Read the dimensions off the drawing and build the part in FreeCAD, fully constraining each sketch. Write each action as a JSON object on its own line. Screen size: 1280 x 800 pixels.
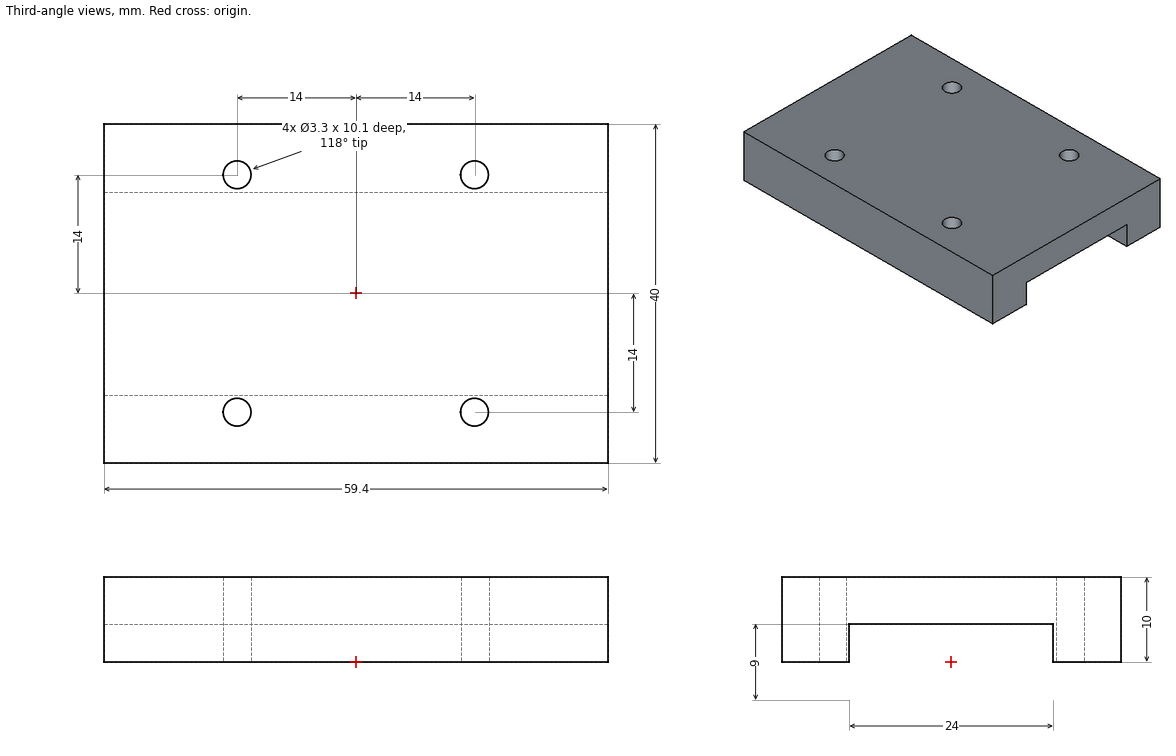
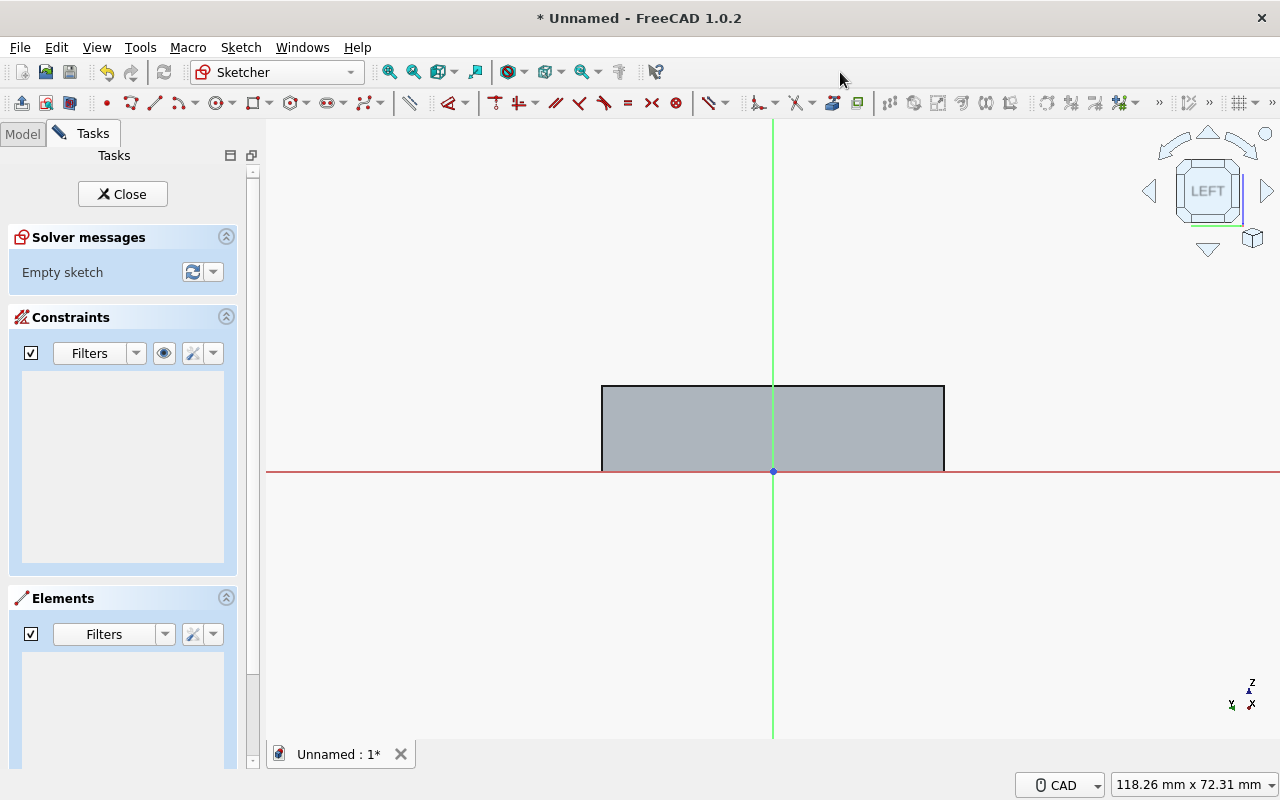
{"action": "scroll", "coordinate": [813, 497], "scroll_direction": "up", "scroll_amount": 5}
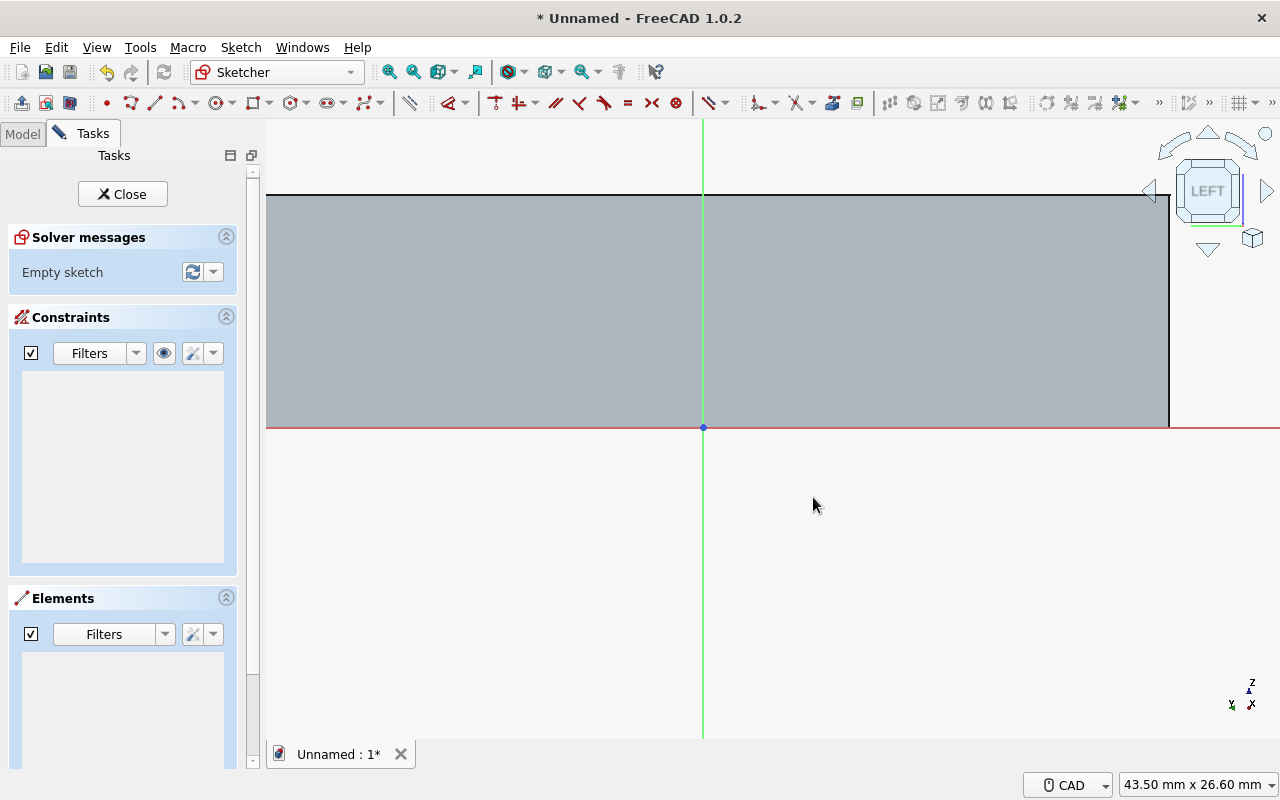
{"action": "key", "text": "g v"}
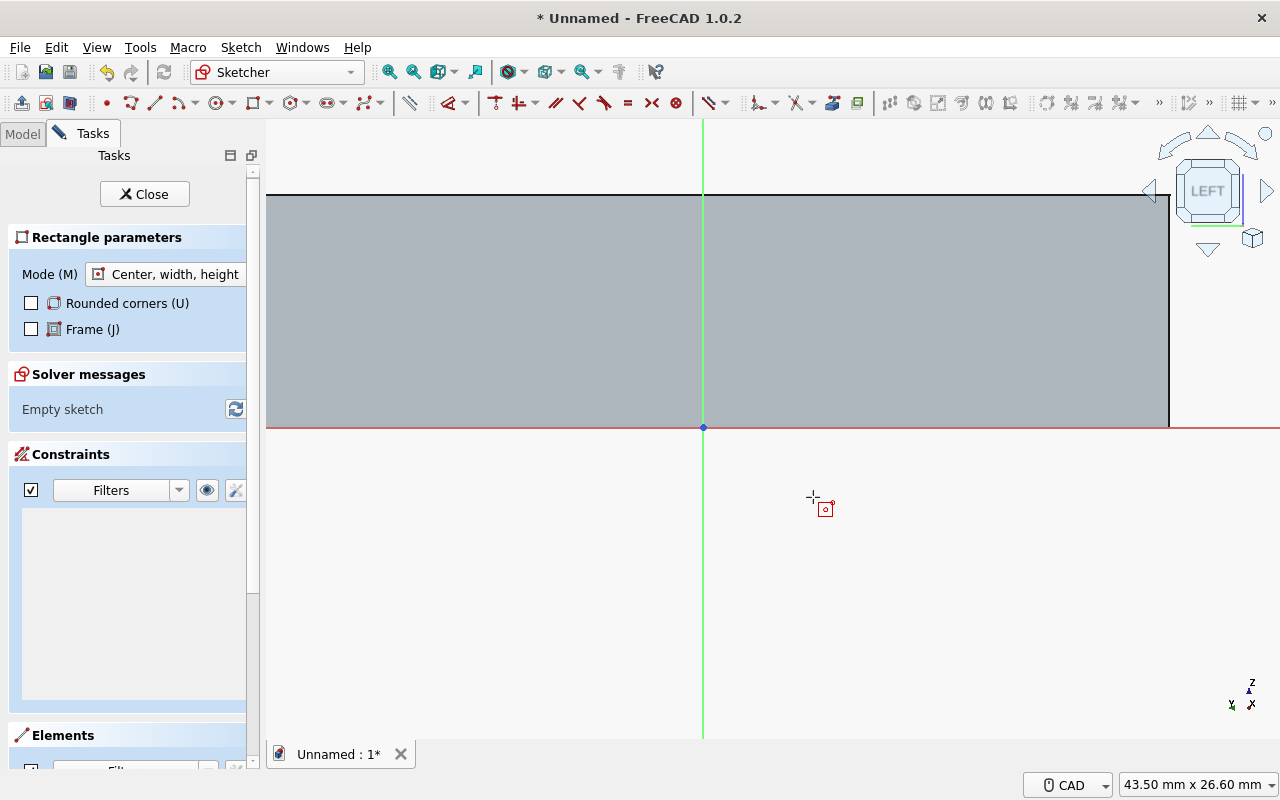
{"action": "left_click", "coordinate": [703, 428]}
{"action": "left_click", "coordinate": [983, 323]}
{"action": "key", "text": "Escape"}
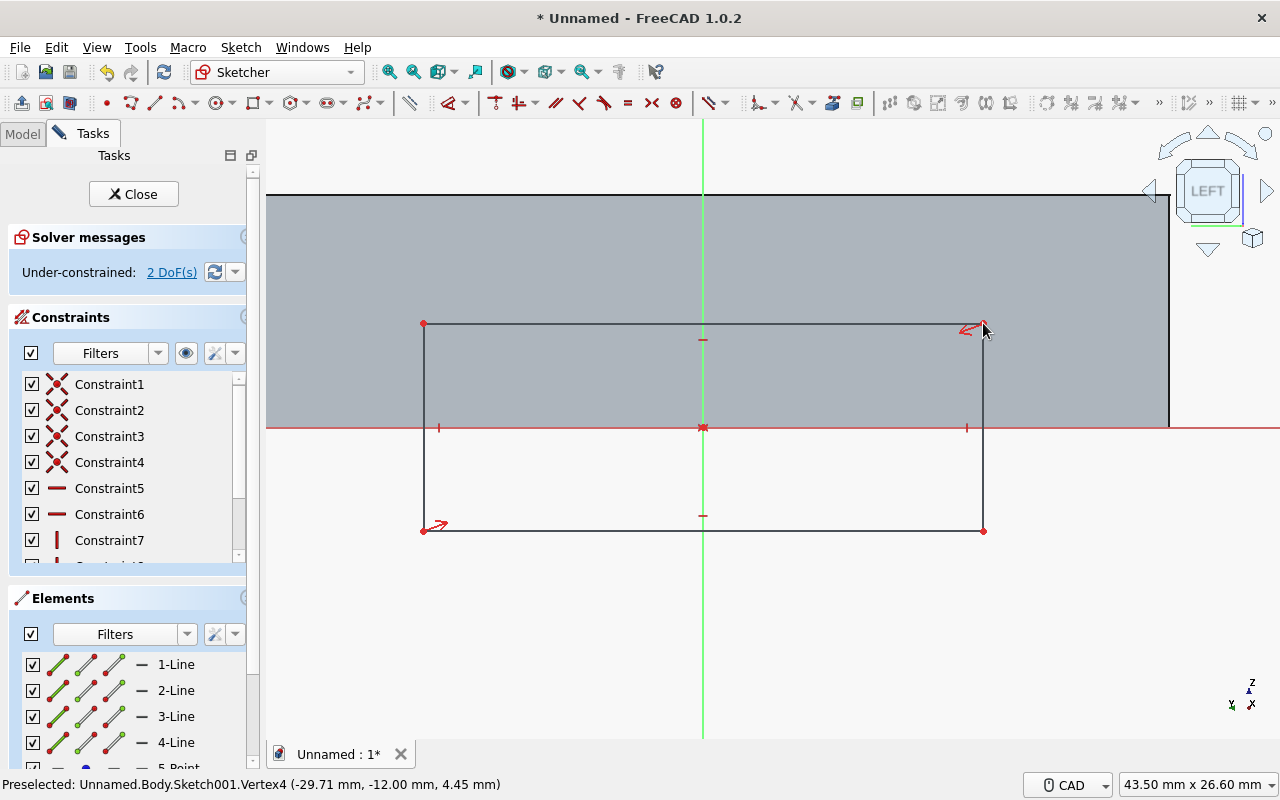
{"action": "key", "text": "d"}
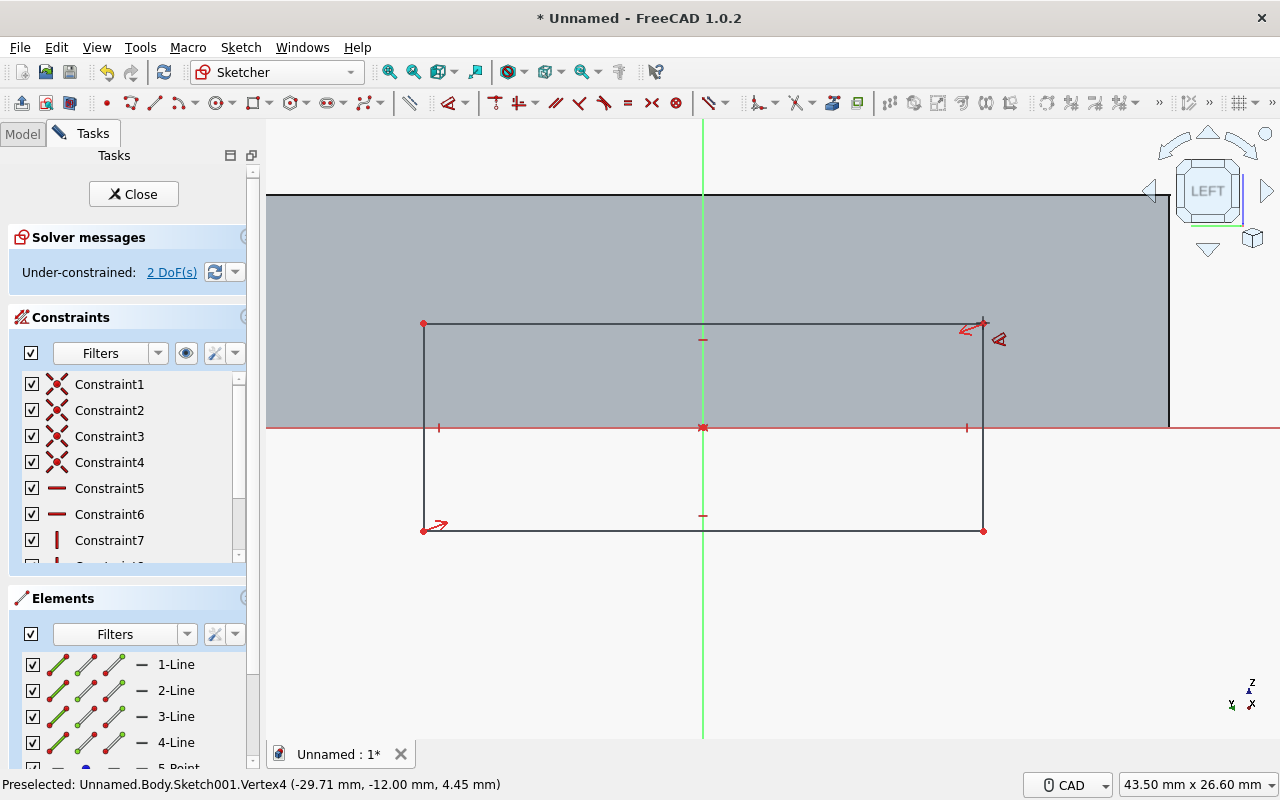
{"action": "left_click", "coordinate": [983, 469]}
{"action": "left_click", "coordinate": [1017, 380]}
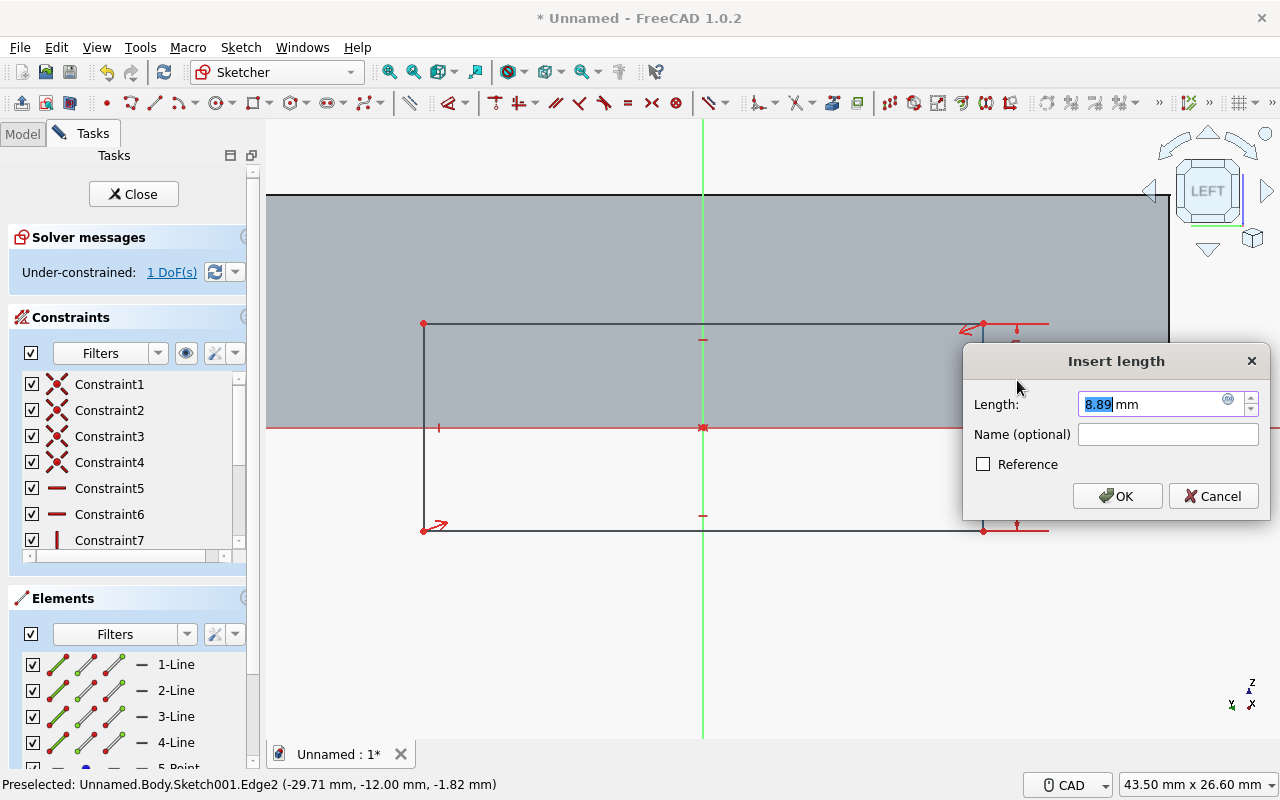
{"action": "type", "text": "9"}
{"action": "key", "text": "Return"}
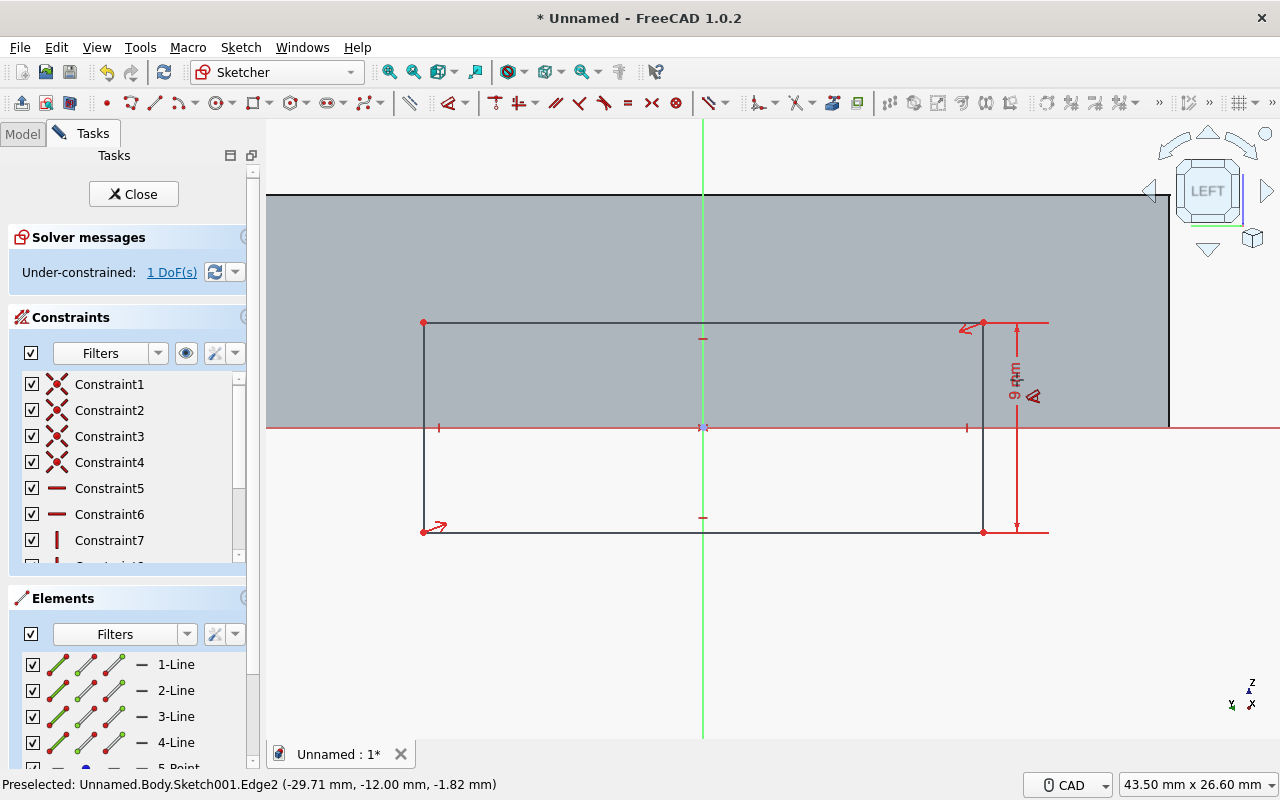
{"action": "left_click", "coordinate": [591, 533]}
{"action": "left_click", "coordinate": [575, 567]}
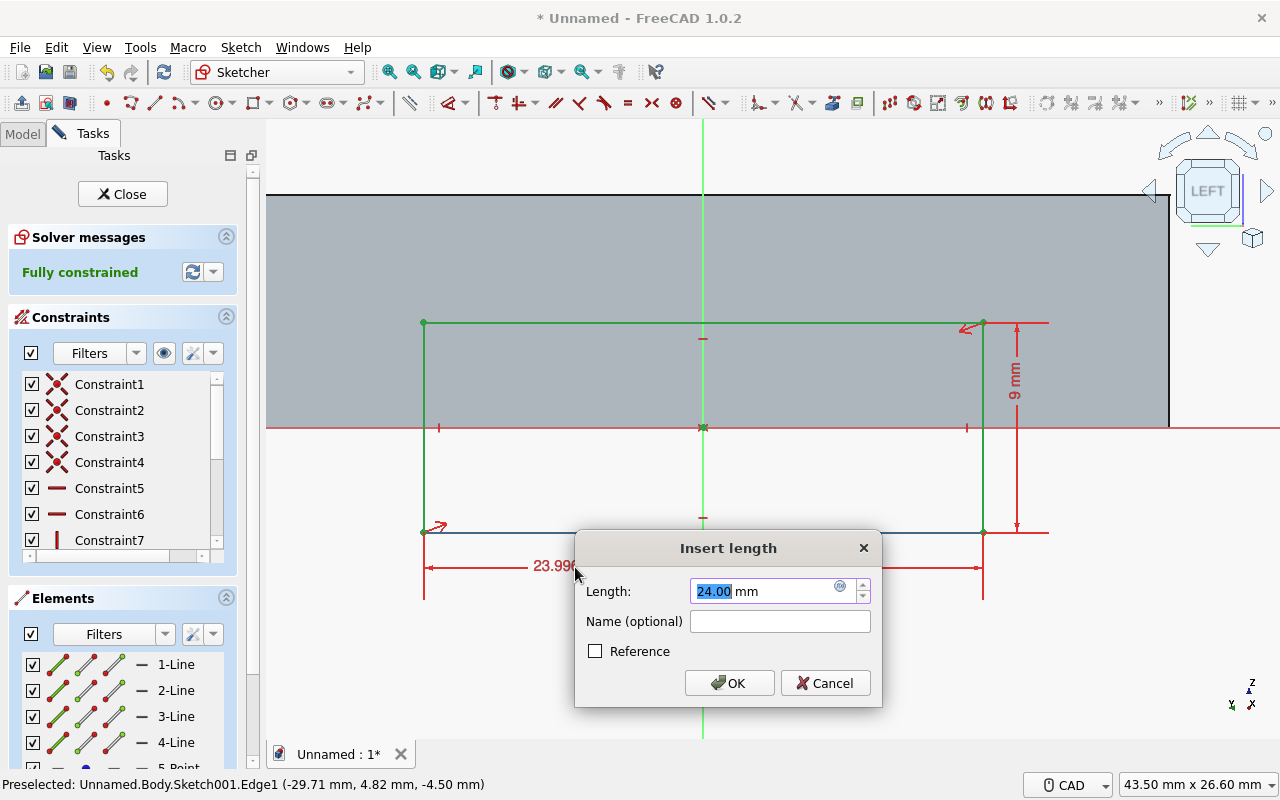
{"action": "type", "text": "24"}
{"action": "key", "text": "Return"}
{"action": "key", "text": "Escape"}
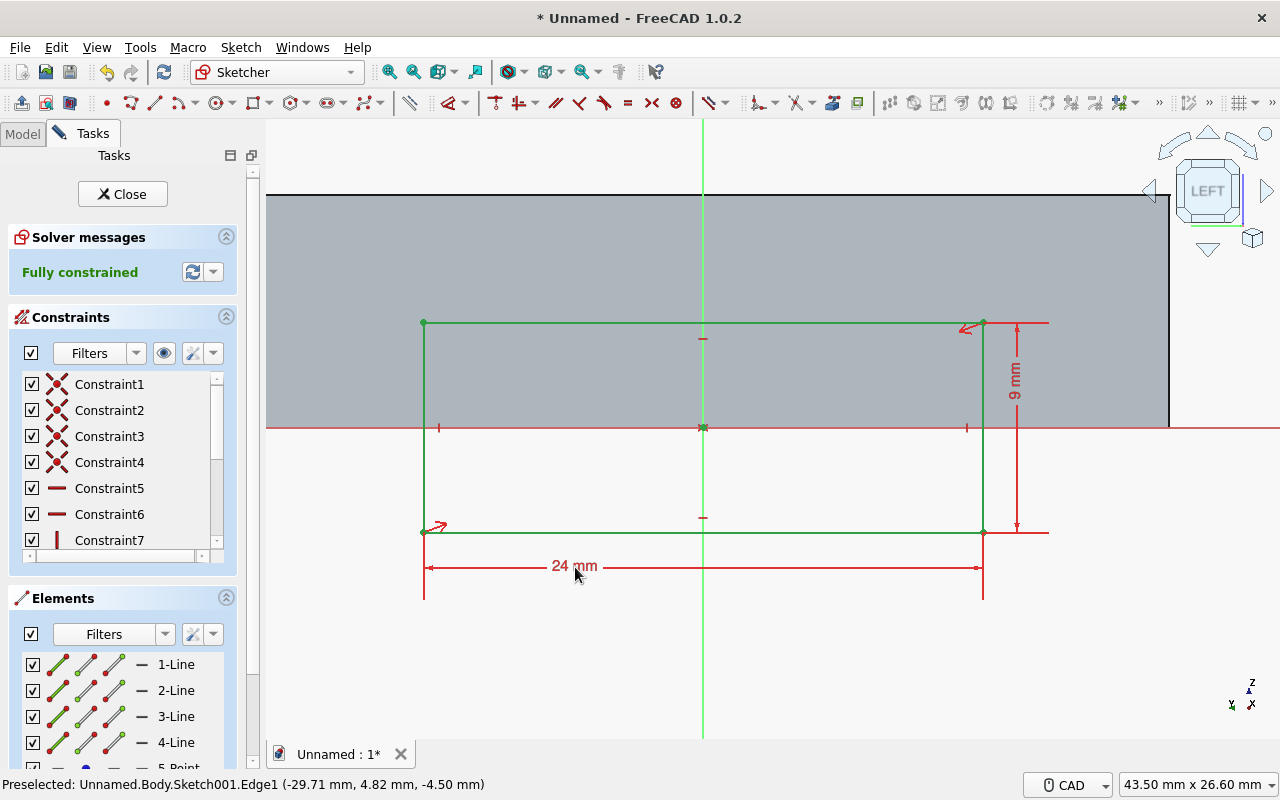
{"action": "left_click", "coordinate": [123, 194]}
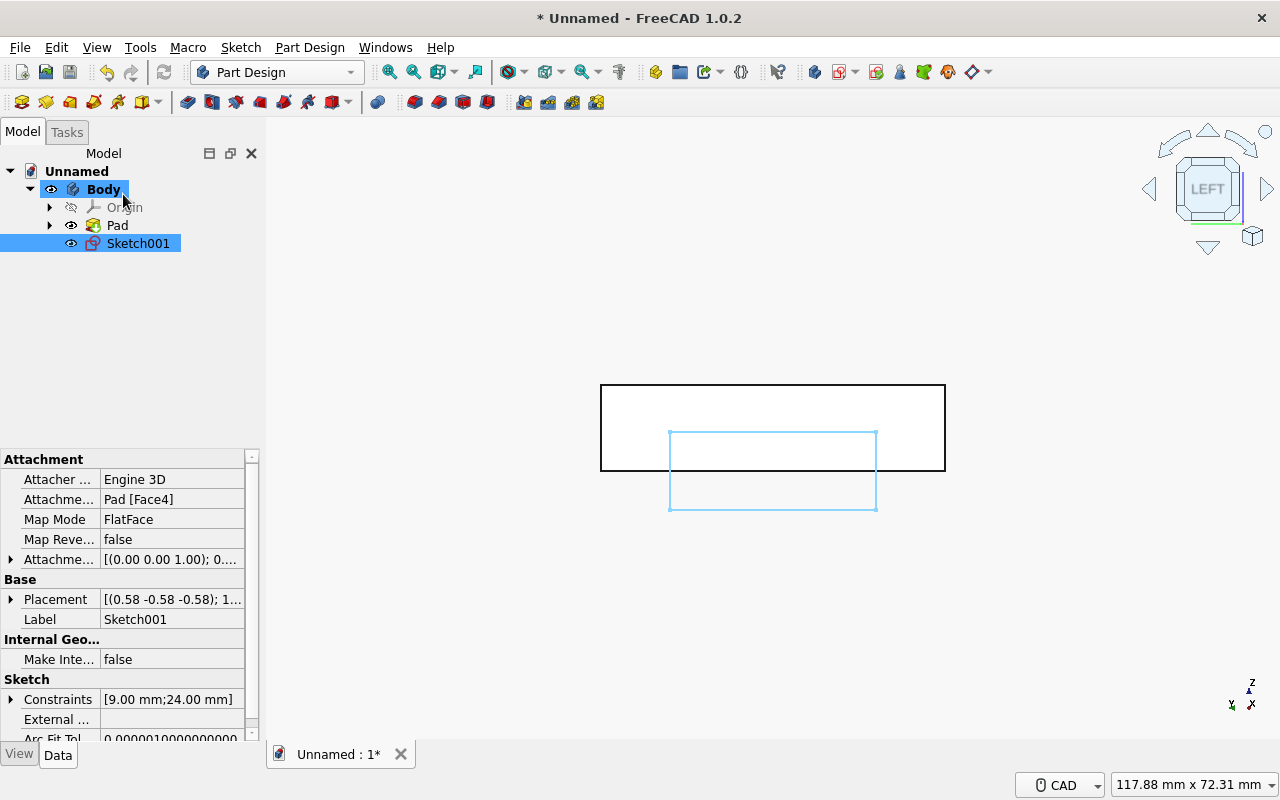
{"action": "left_click", "coordinate": [188, 102]}